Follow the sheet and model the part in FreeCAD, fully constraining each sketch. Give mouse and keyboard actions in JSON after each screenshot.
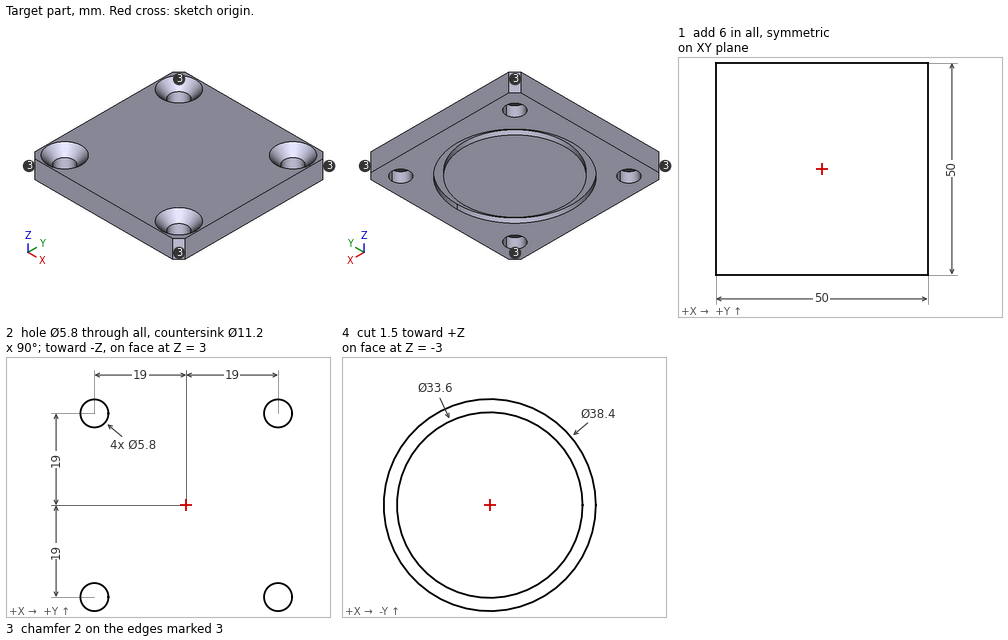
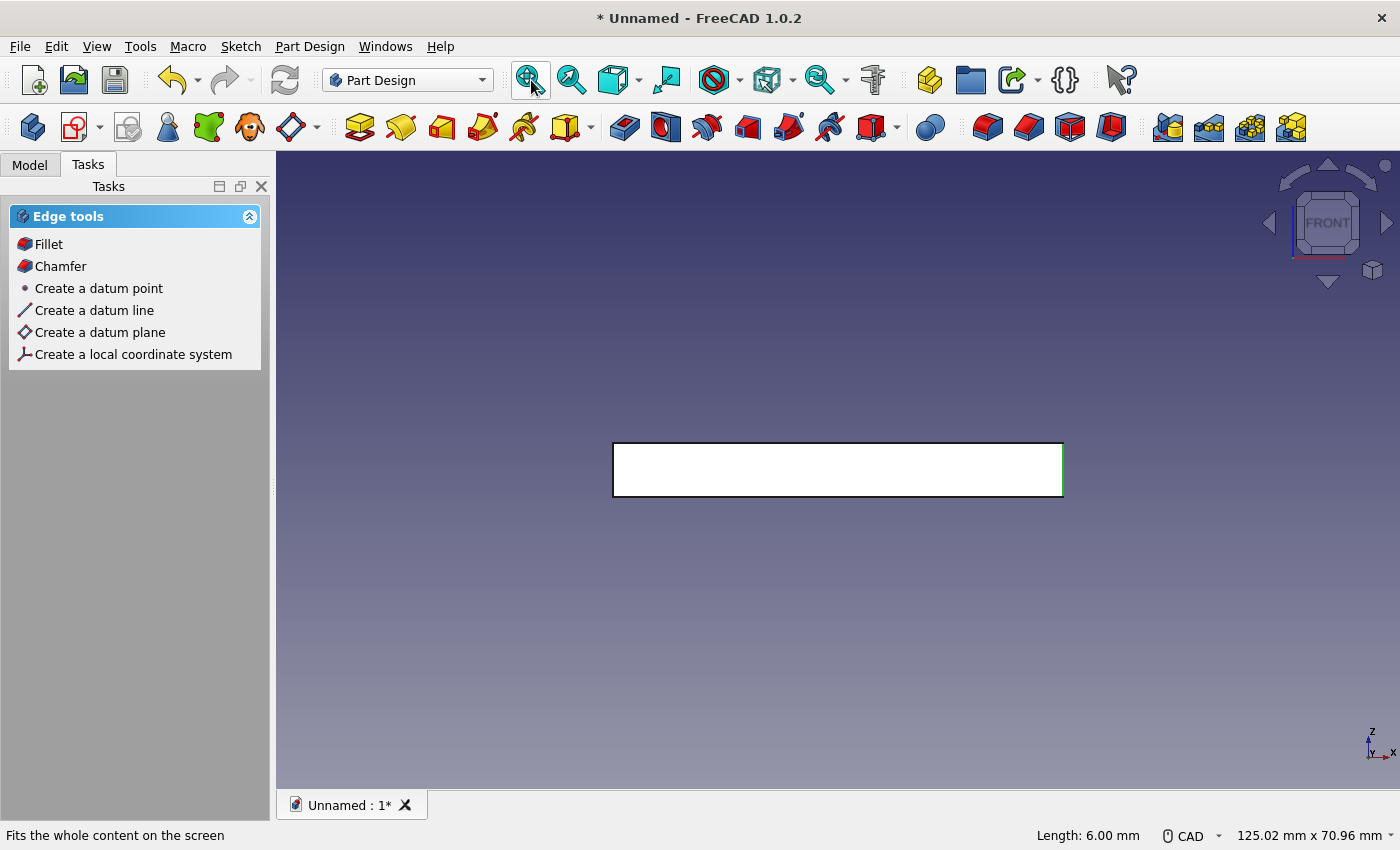
{"action": "left_click", "coordinate": [613, 469], "text": "ctrl"}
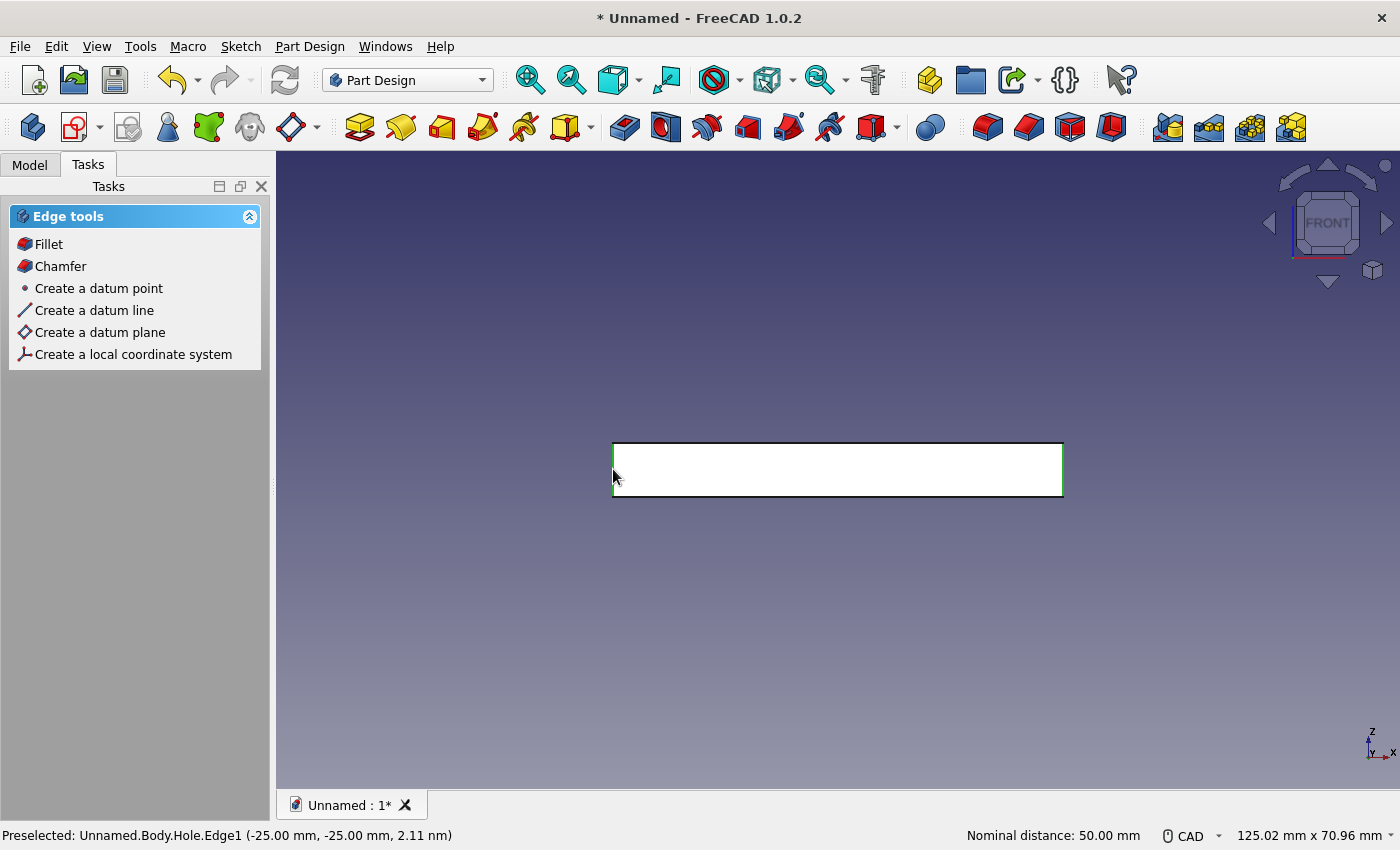
{"action": "key", "text": "3"}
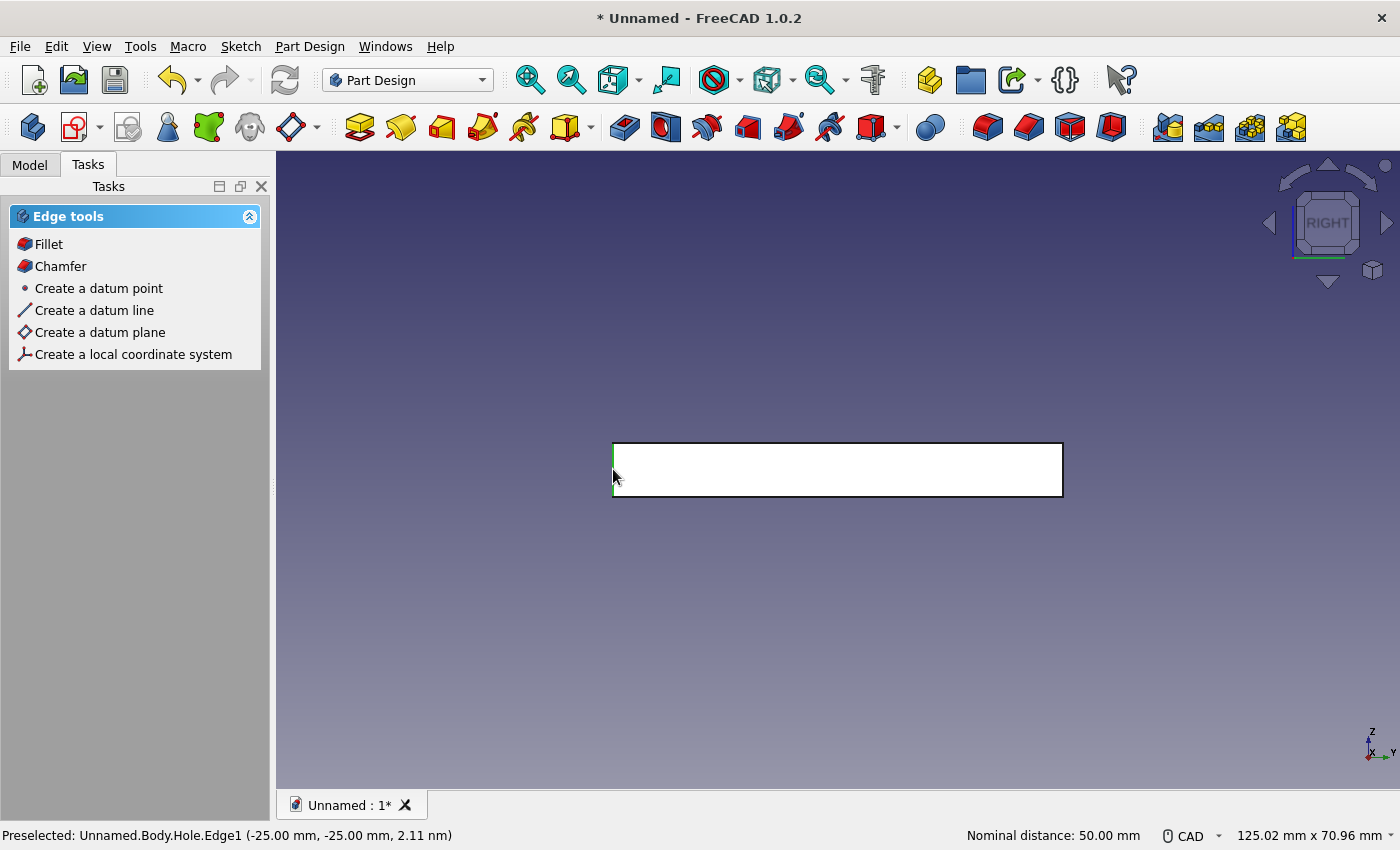
{"action": "left_click", "coordinate": [531, 80]}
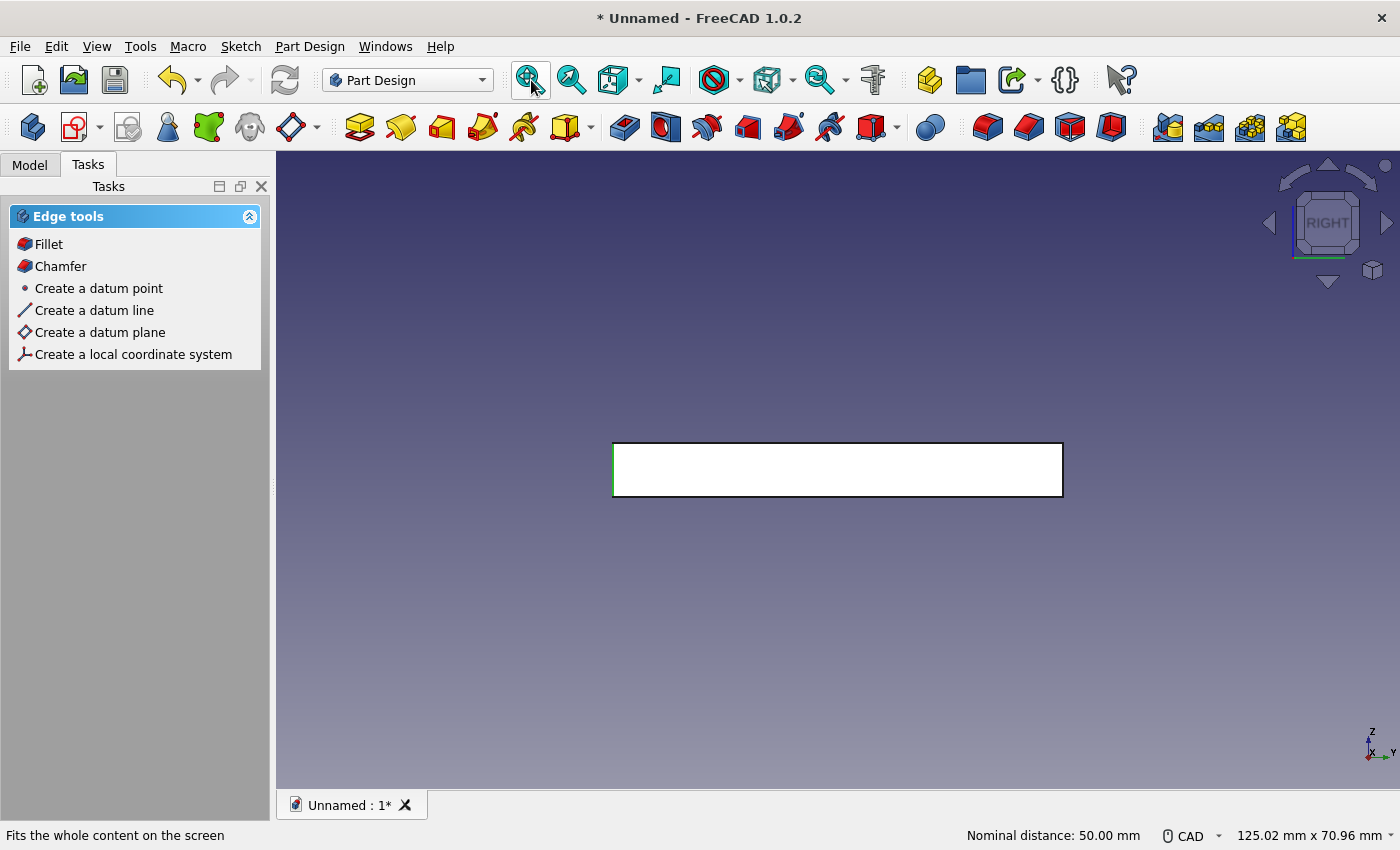
{"action": "left_click", "coordinate": [1063, 469], "text": "ctrl"}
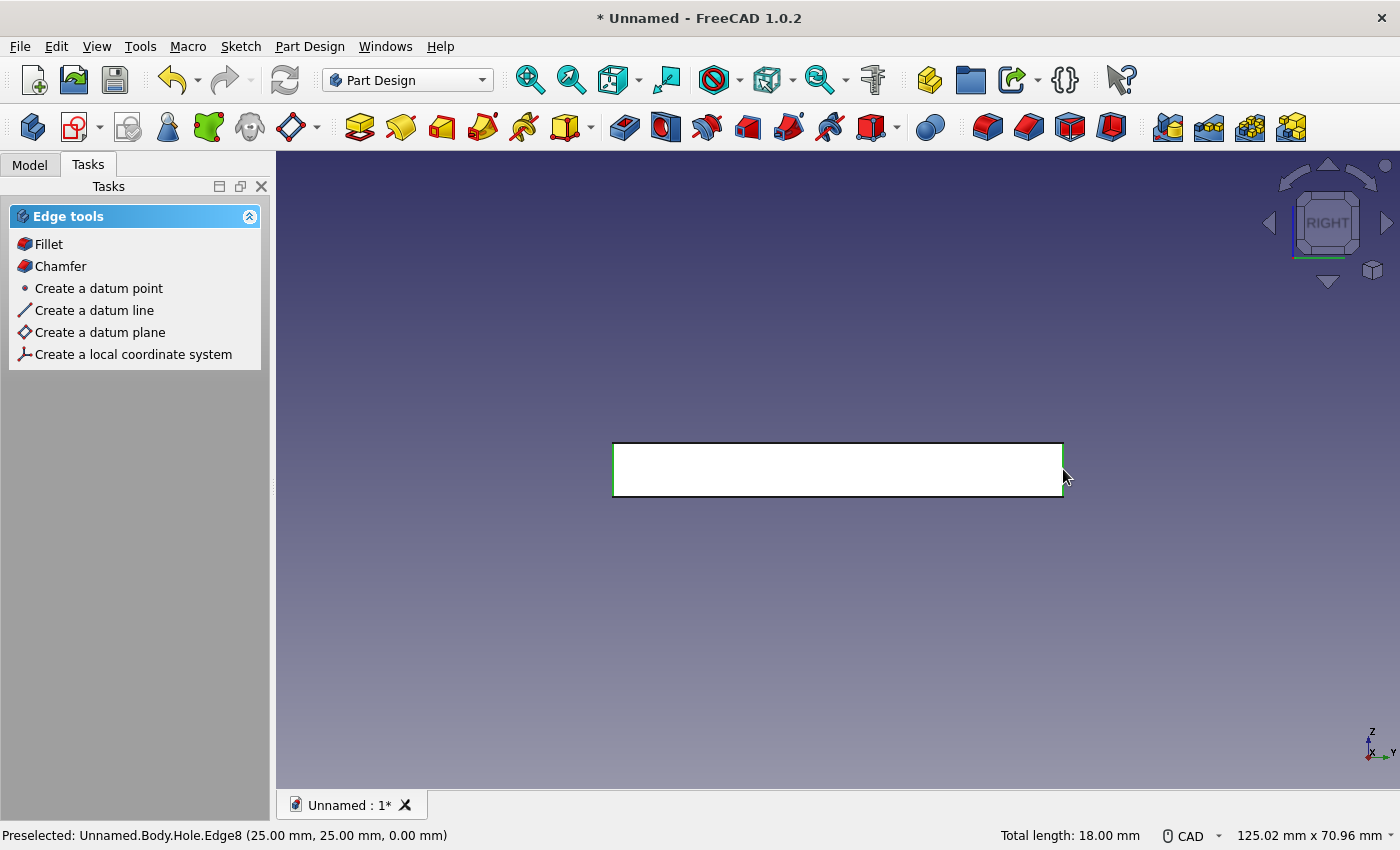
{"action": "key", "text": "5"}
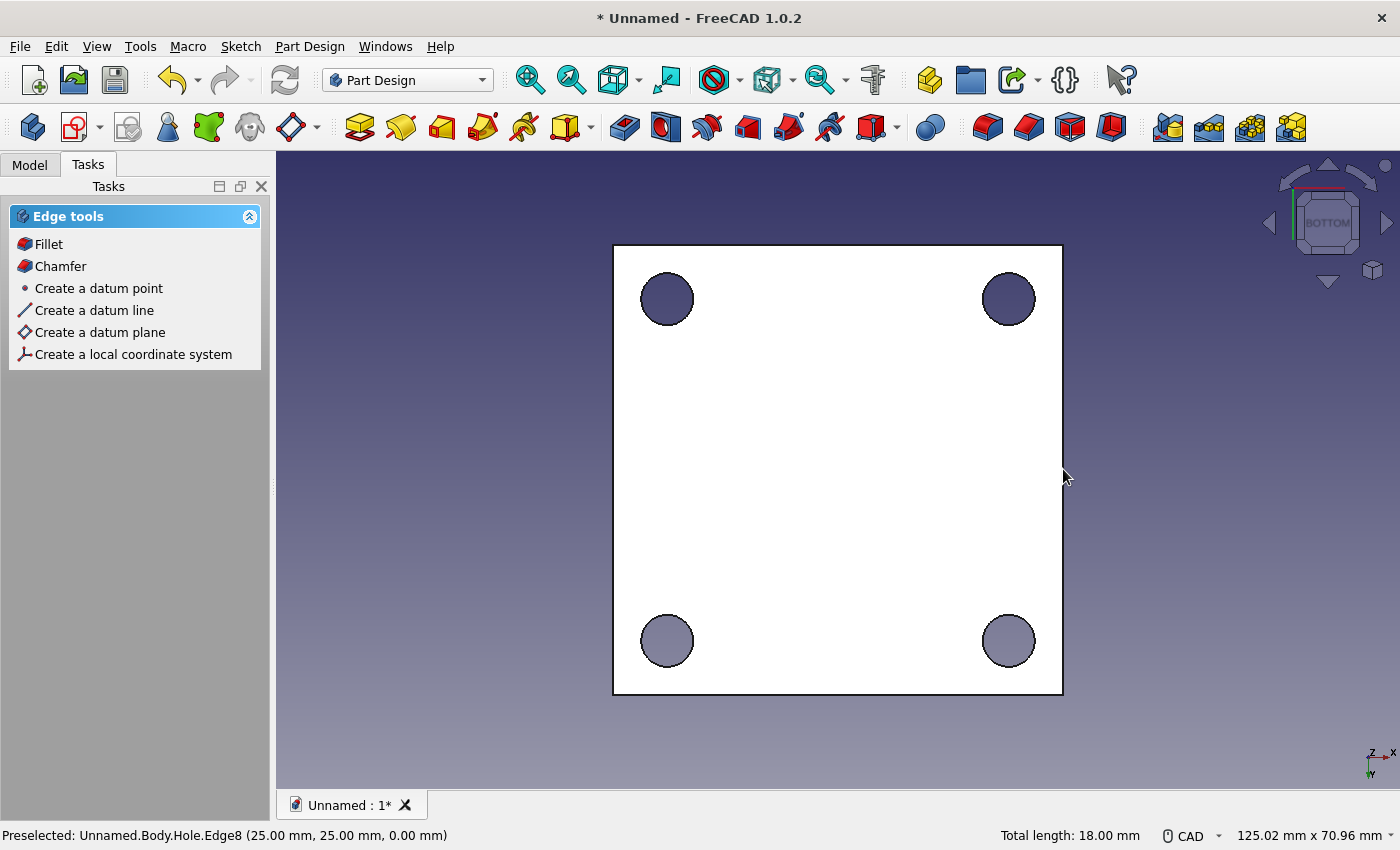
{"action": "key", "text": "4"}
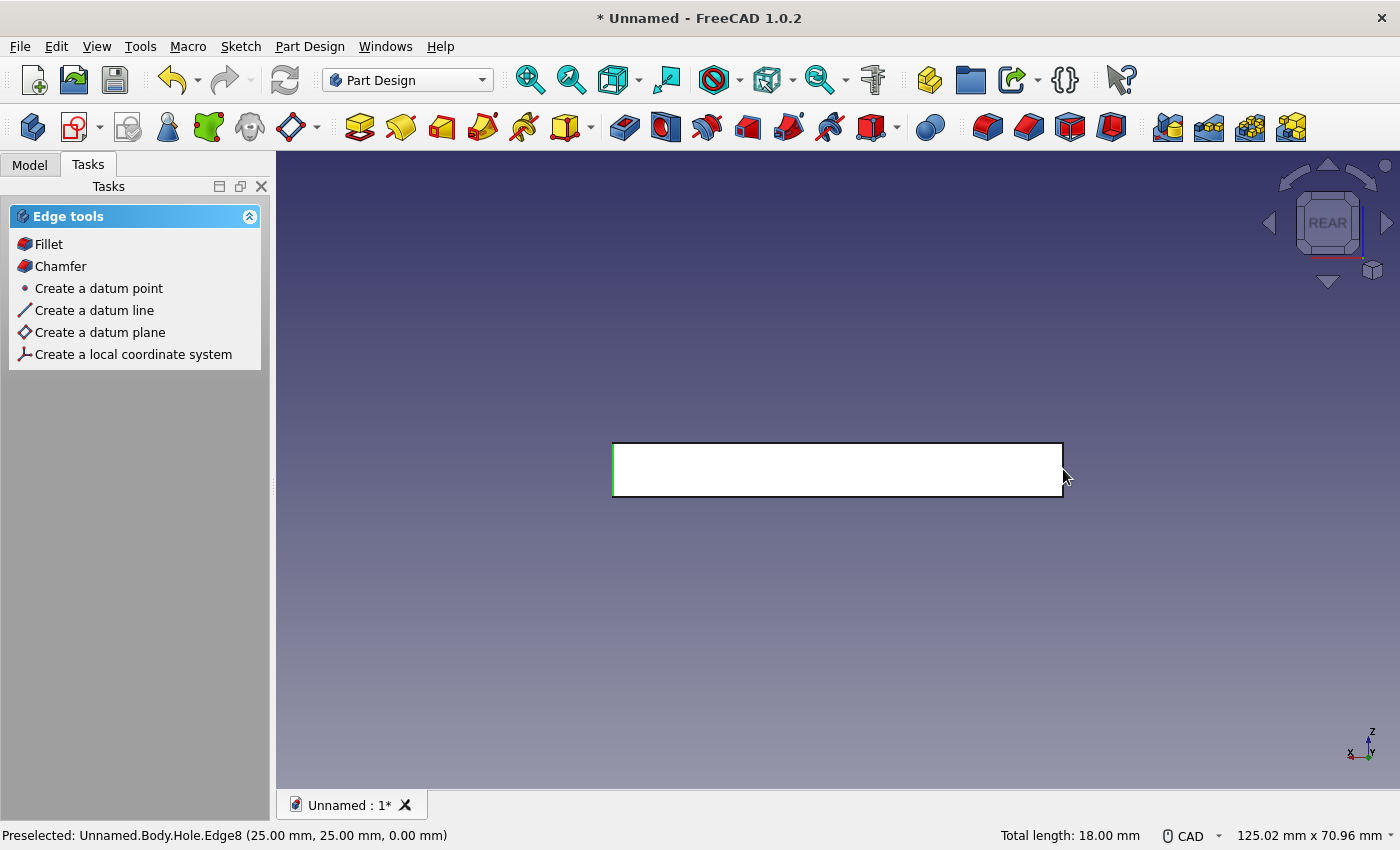
{"action": "left_click", "coordinate": [531, 80]}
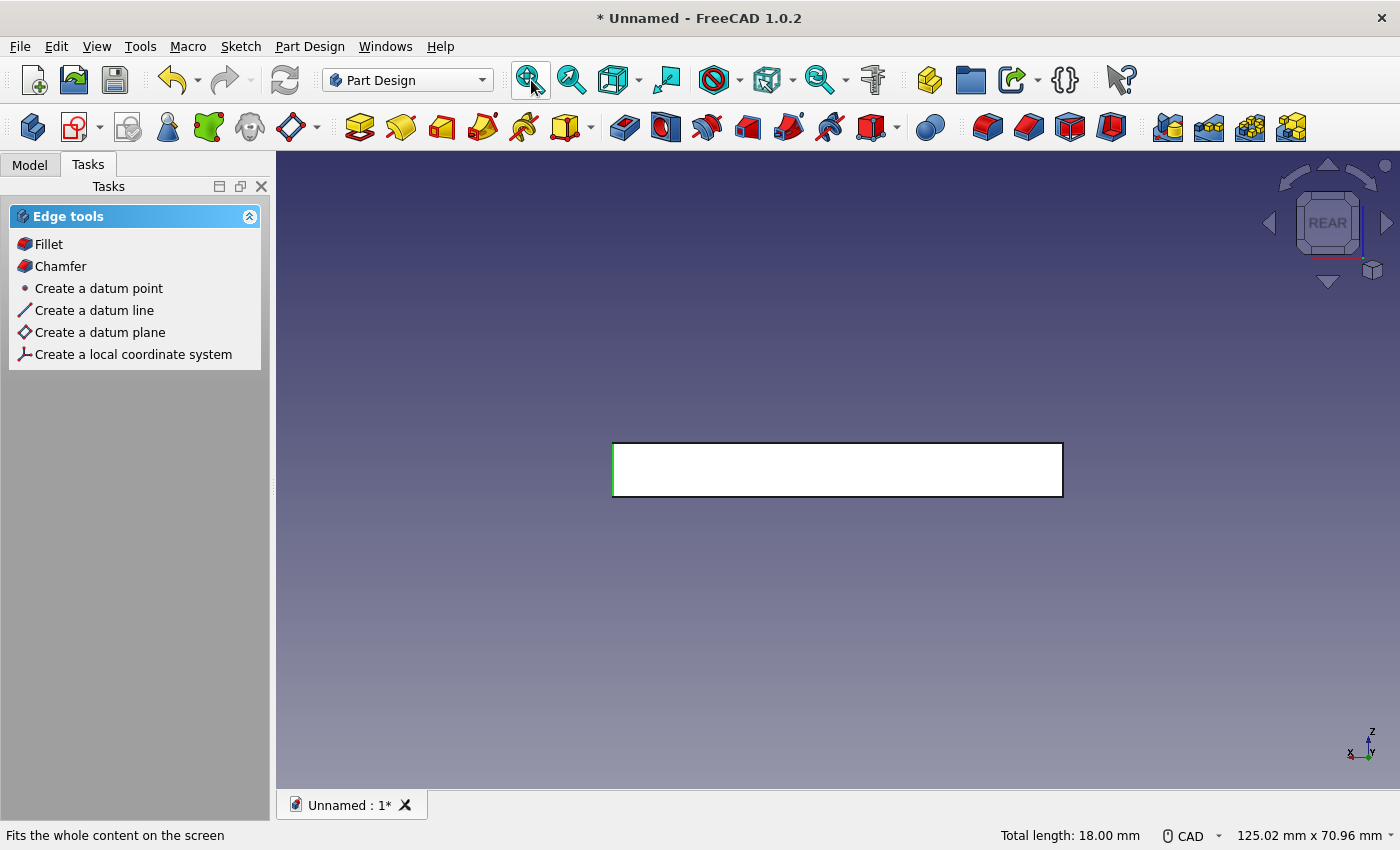
{"action": "left_click", "coordinate": [1063, 469], "text": "ctrl"}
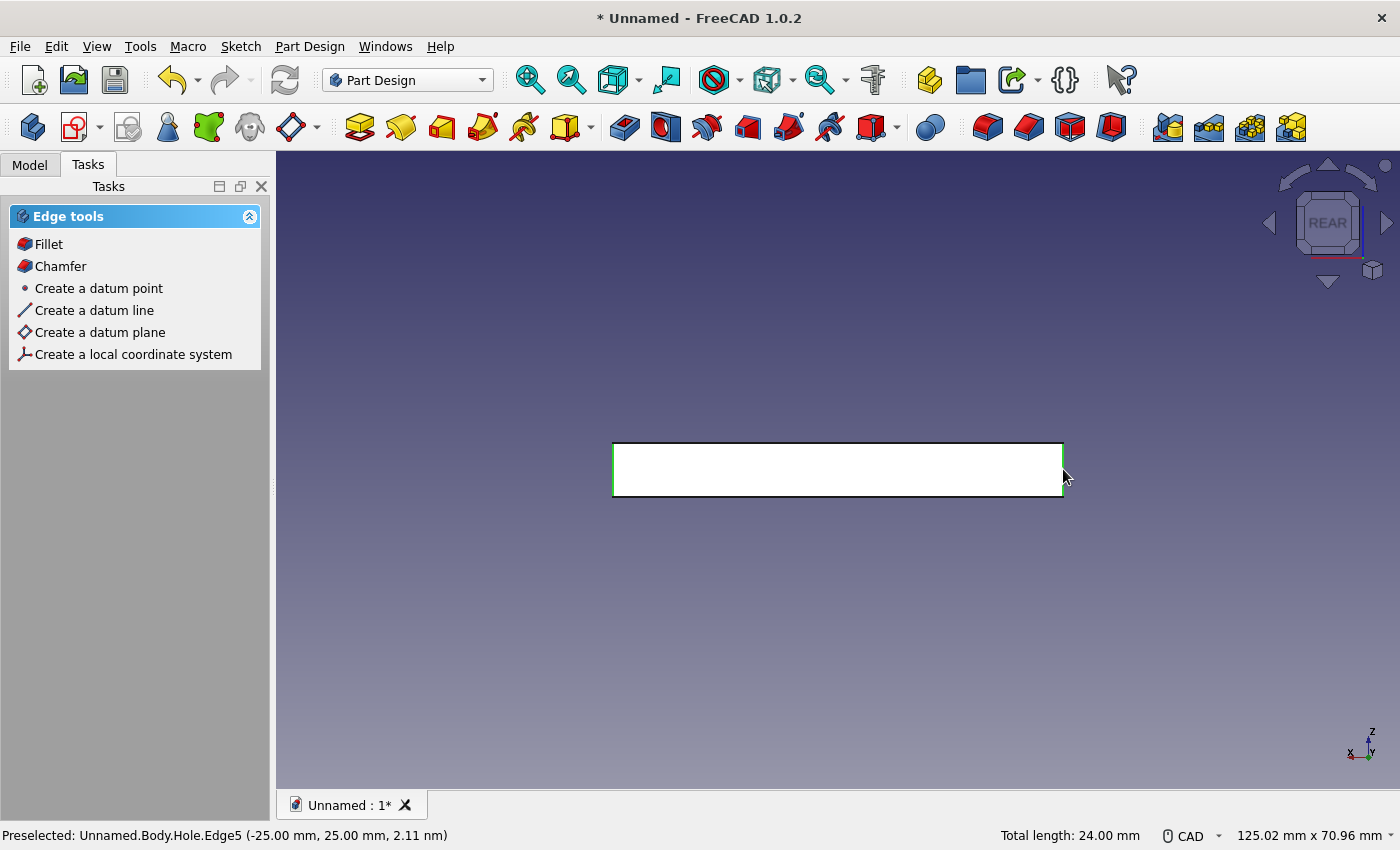
{"action": "left_click", "coordinate": [1029, 128]}